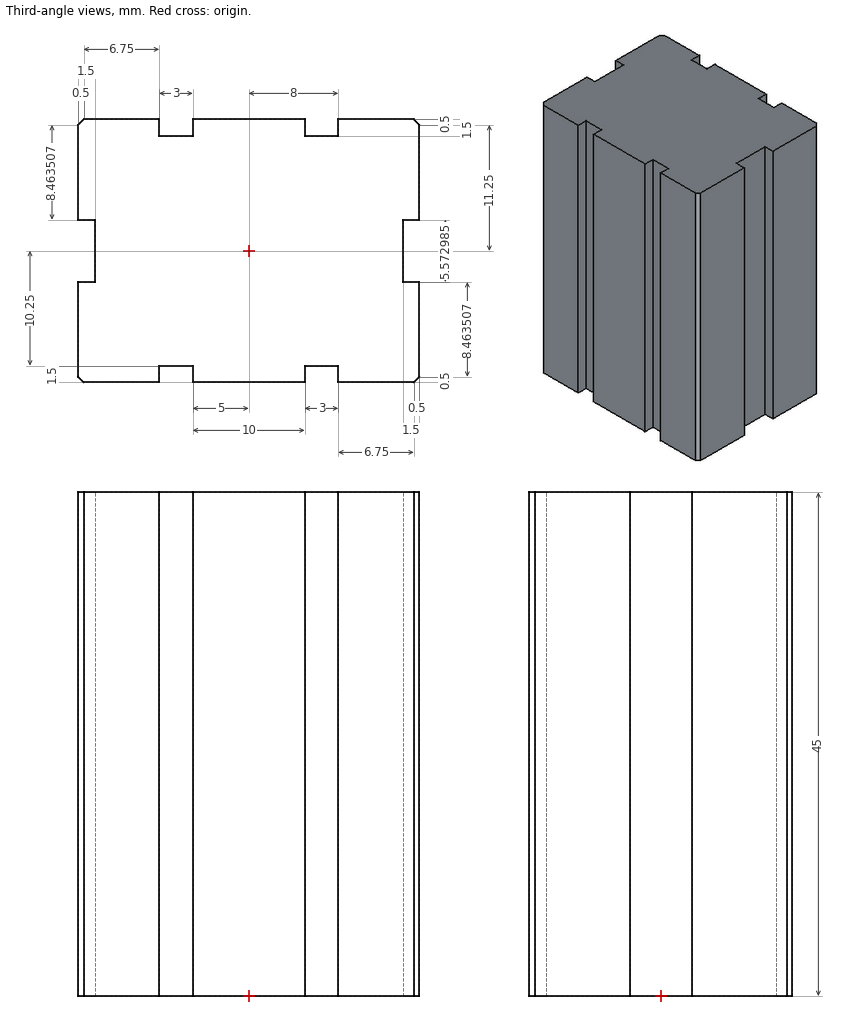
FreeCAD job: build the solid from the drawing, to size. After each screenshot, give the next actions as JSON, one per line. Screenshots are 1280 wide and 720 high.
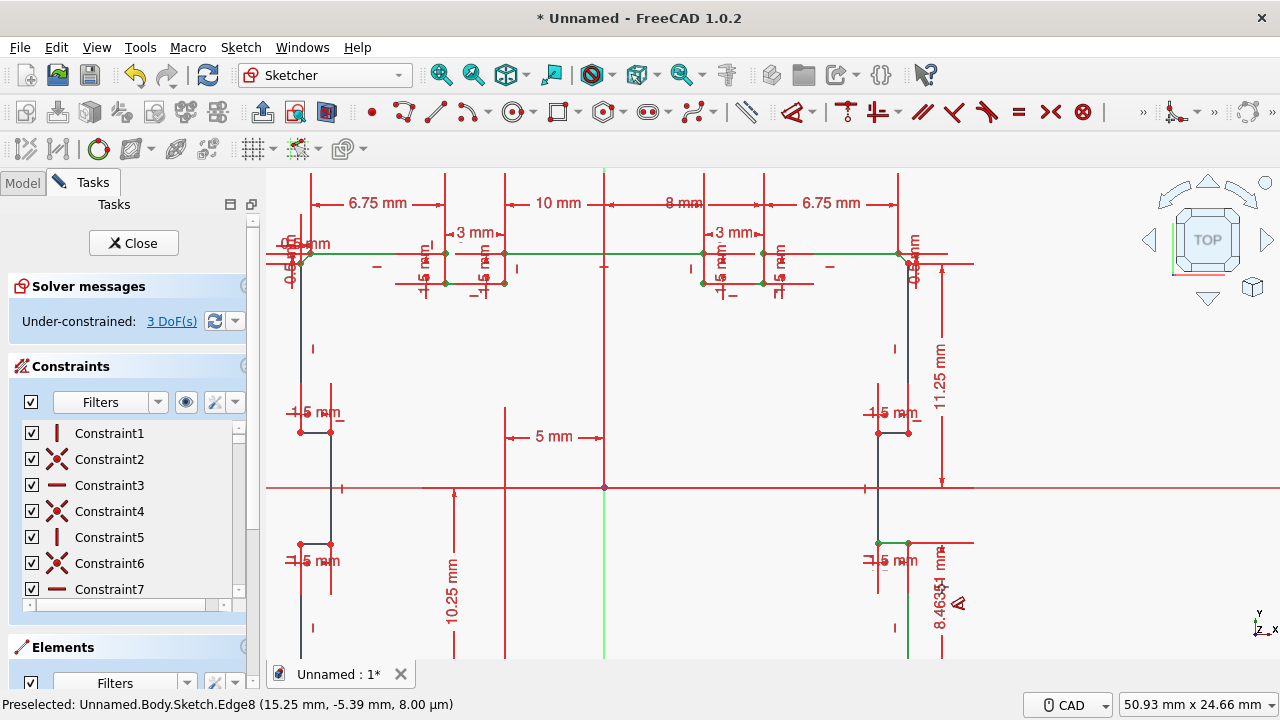
{"action": "left_click", "coordinate": [878, 510]}
{"action": "left_click", "coordinate": [912, 463]}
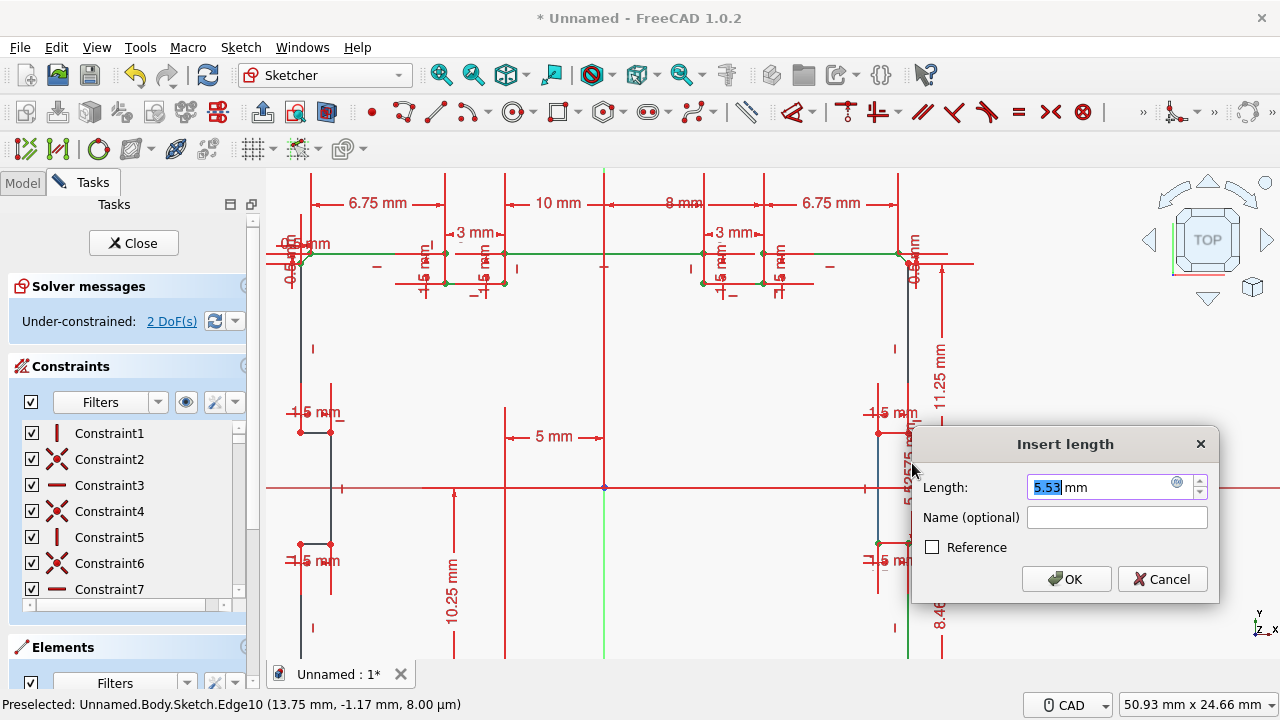
{"action": "type", "text": "5.572985"}
{"action": "key", "text": "Return"}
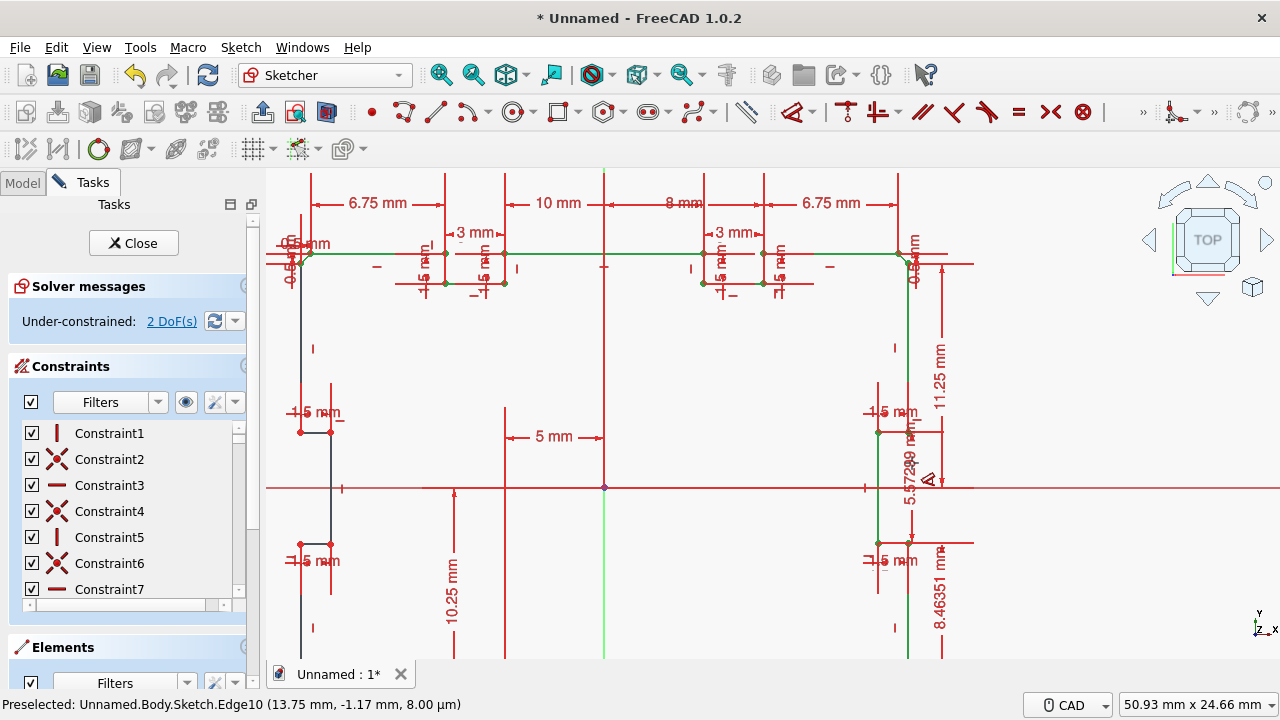
{"action": "left_click", "coordinate": [301, 314]}
{"action": "left_click", "coordinate": [335, 348]}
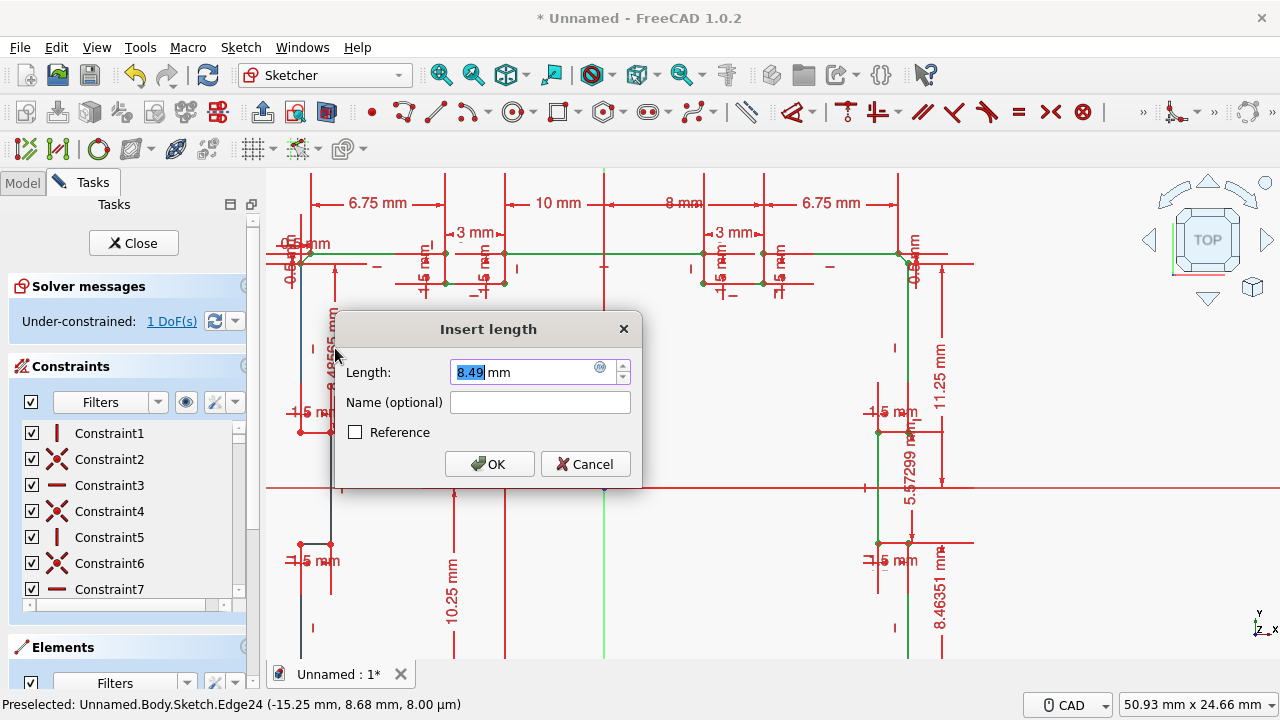
{"action": "type", "text": "8.463507"}
{"action": "key", "text": "Return"}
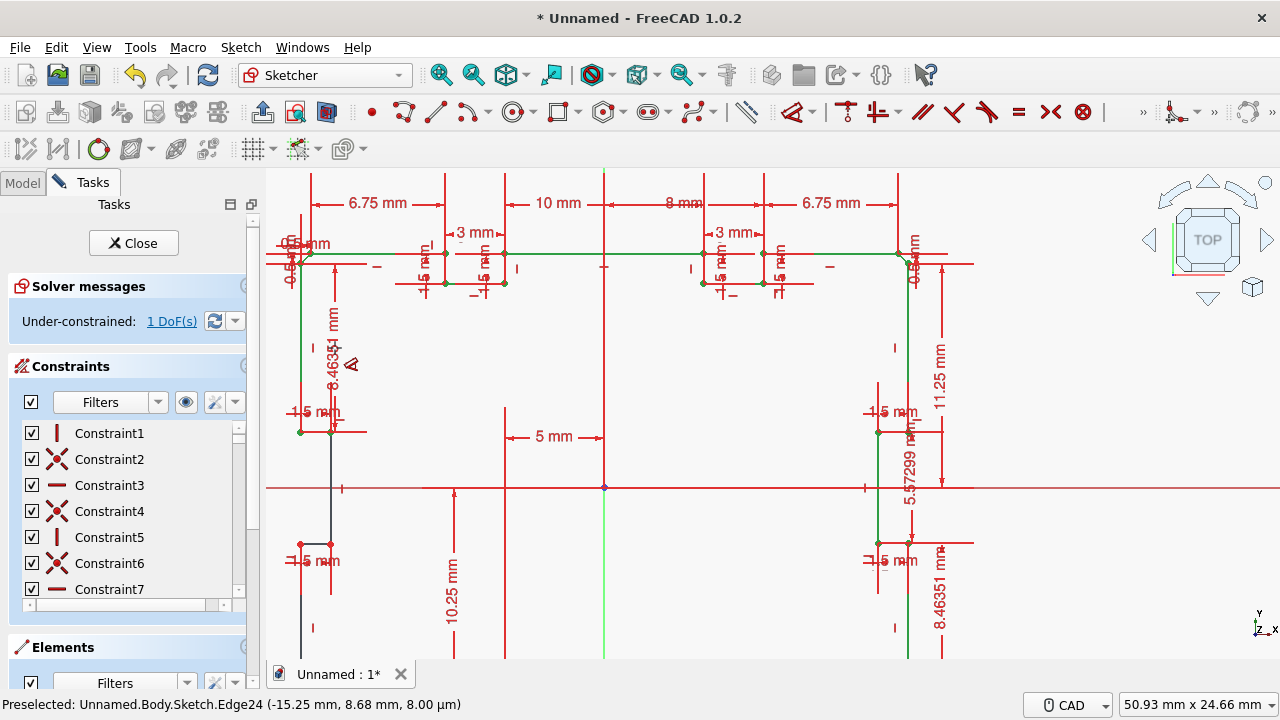
{"action": "left_click", "coordinate": [331, 466]}
{"action": "left_click", "coordinate": [297, 462]}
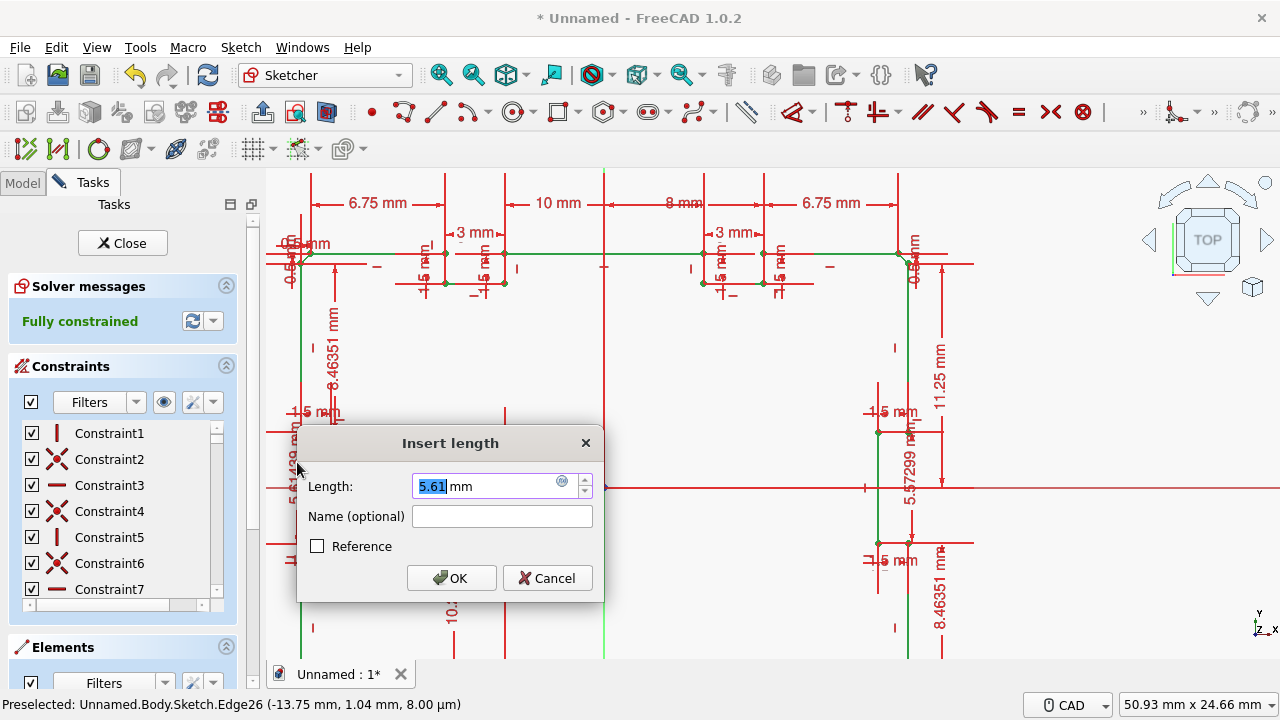
{"action": "type", "text": "5.572985"}
{"action": "key", "text": "Return"}
{"action": "key", "text": "Escape"}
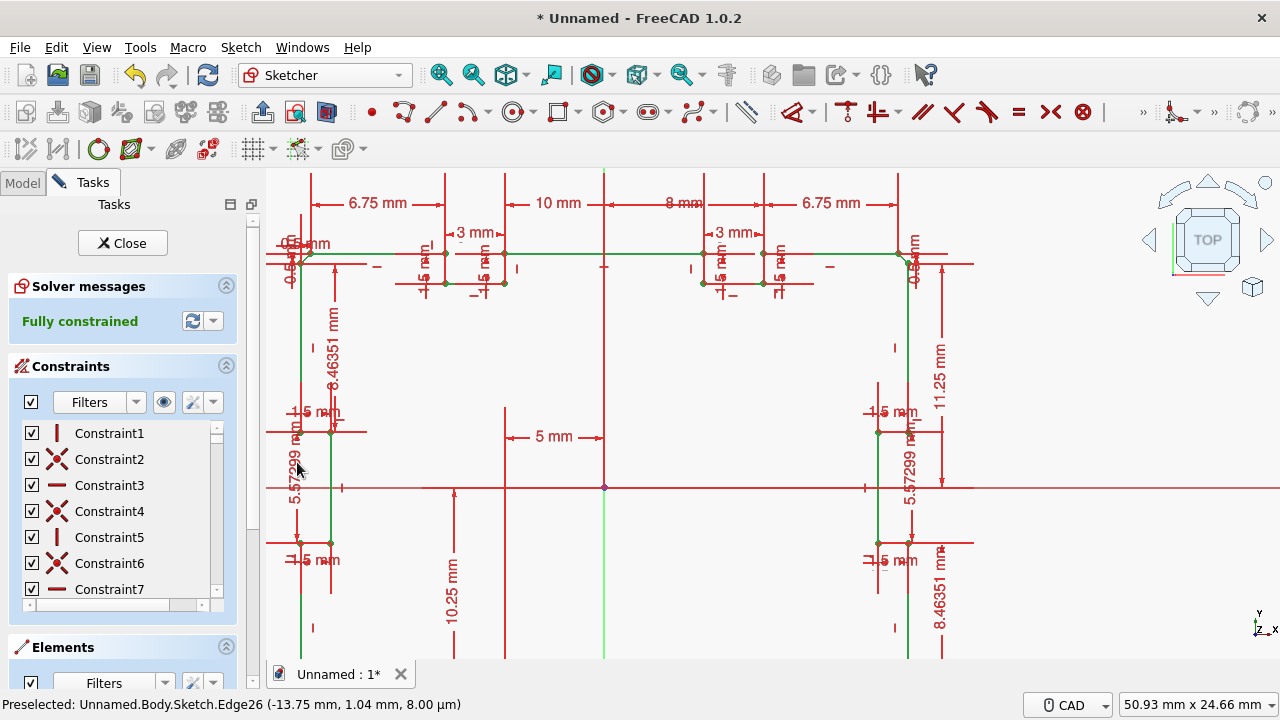
{"action": "left_click", "coordinate": [123, 243]}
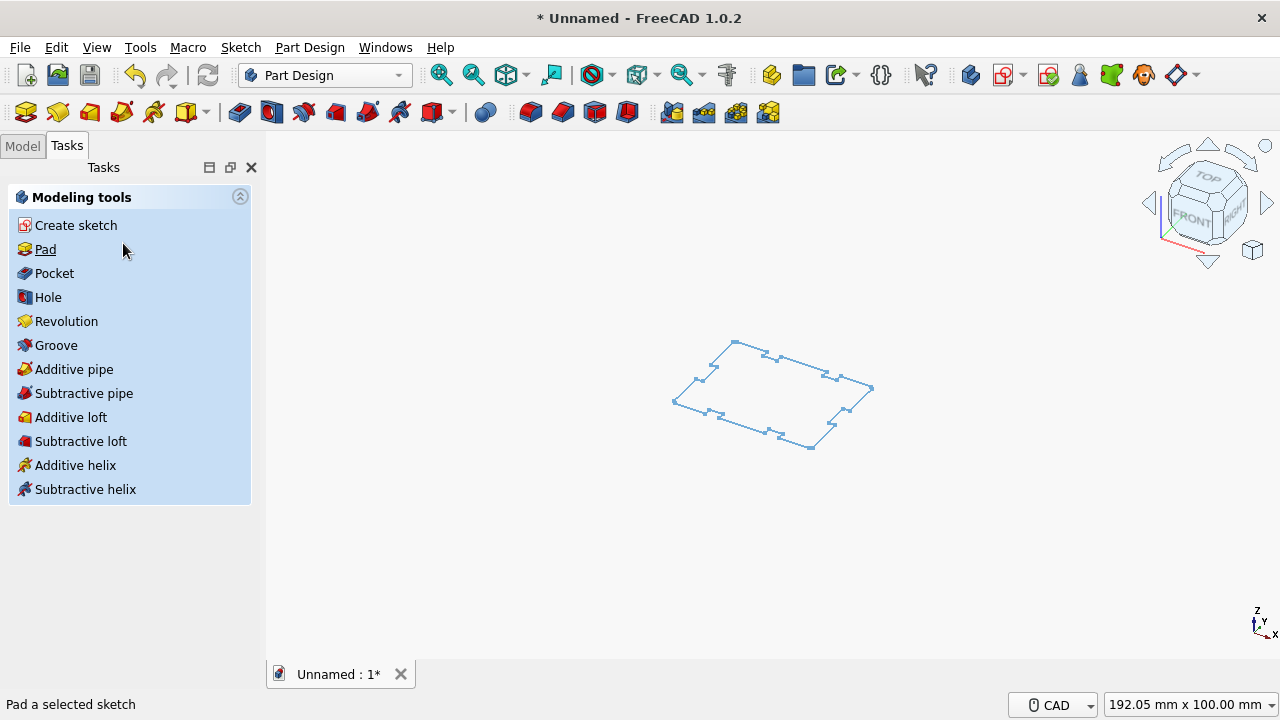
{"action": "left_click", "coordinate": [26, 112]}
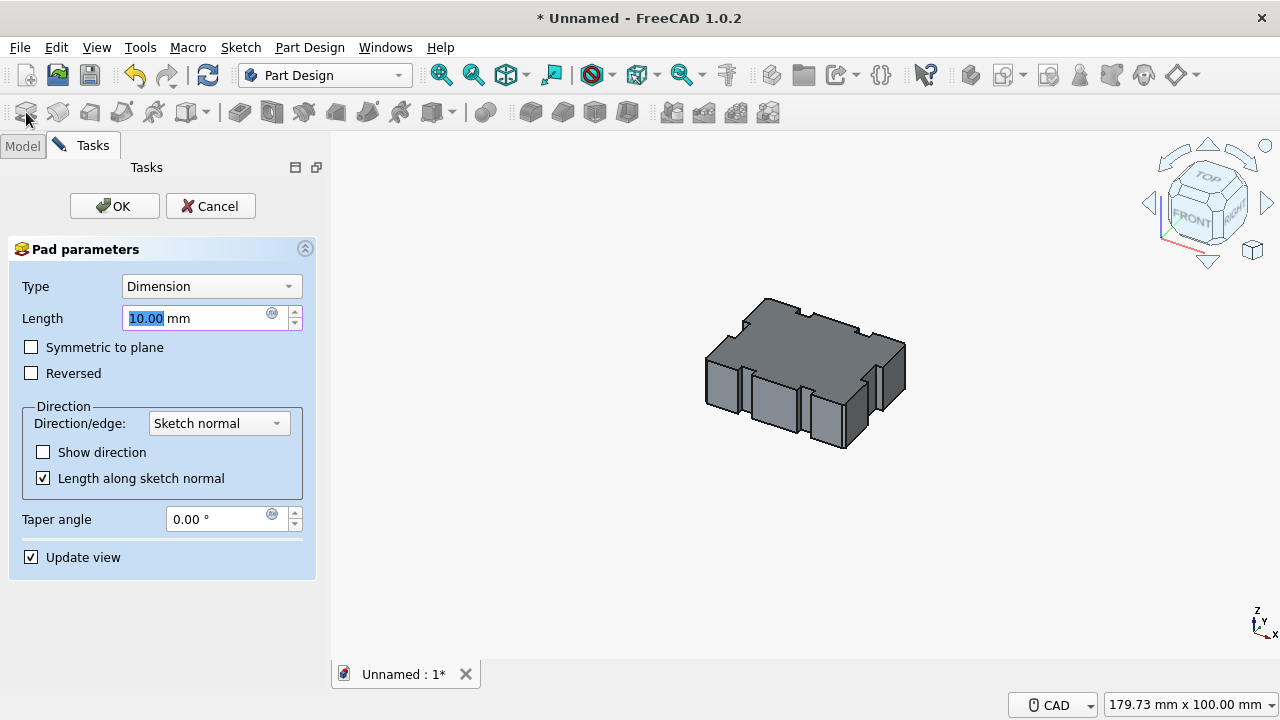
{"action": "type", "text": "45"}
{"action": "key", "text": "Tab"}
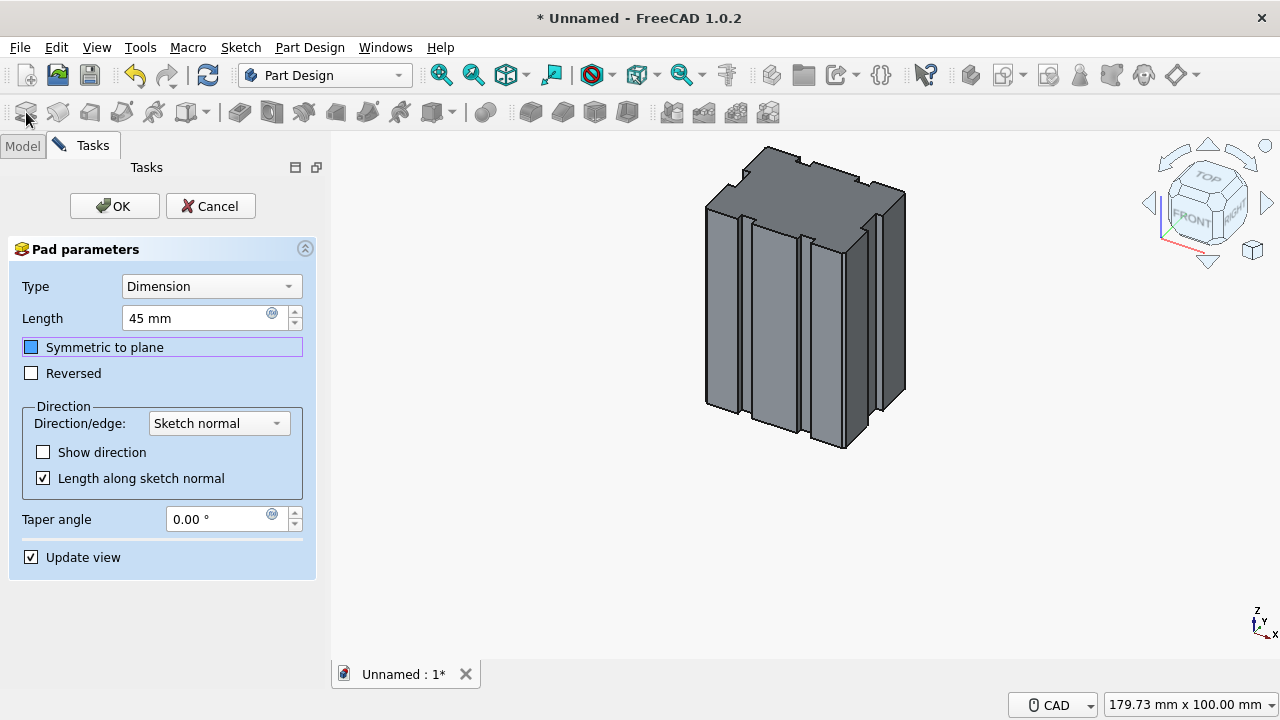
{"action": "left_click", "coordinate": [115, 206]}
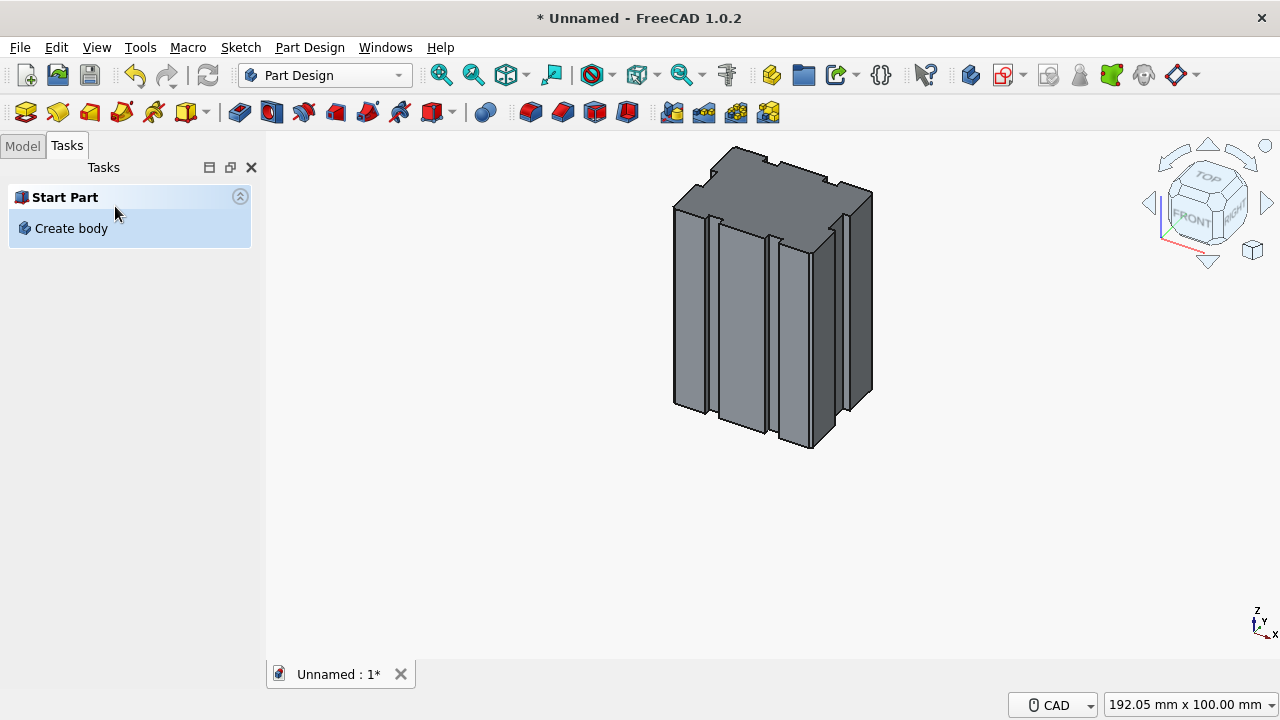
{"action": "key", "text": "0"}